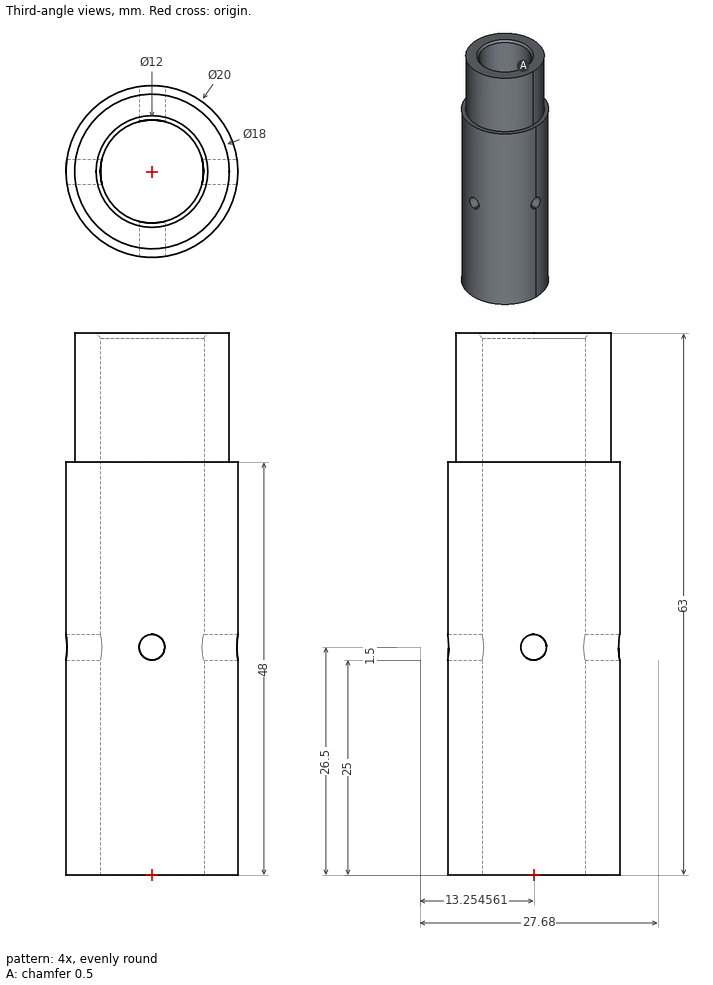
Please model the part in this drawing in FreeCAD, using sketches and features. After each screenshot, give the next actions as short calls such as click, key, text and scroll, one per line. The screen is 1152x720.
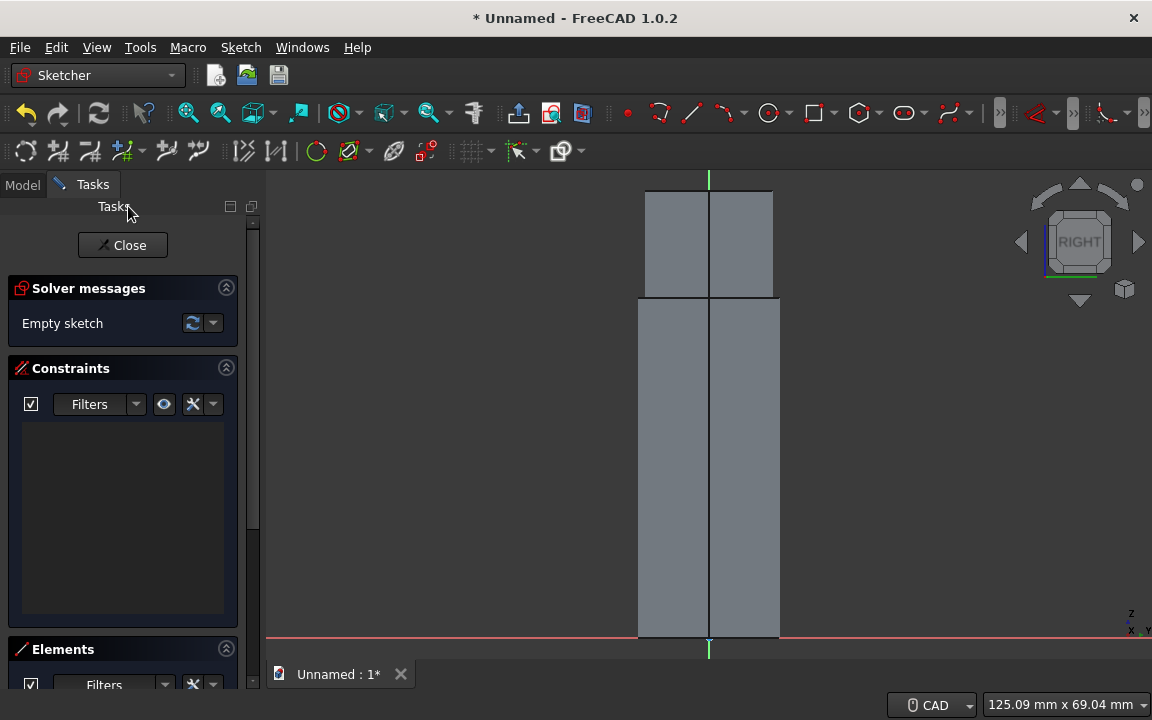
click(584, 114)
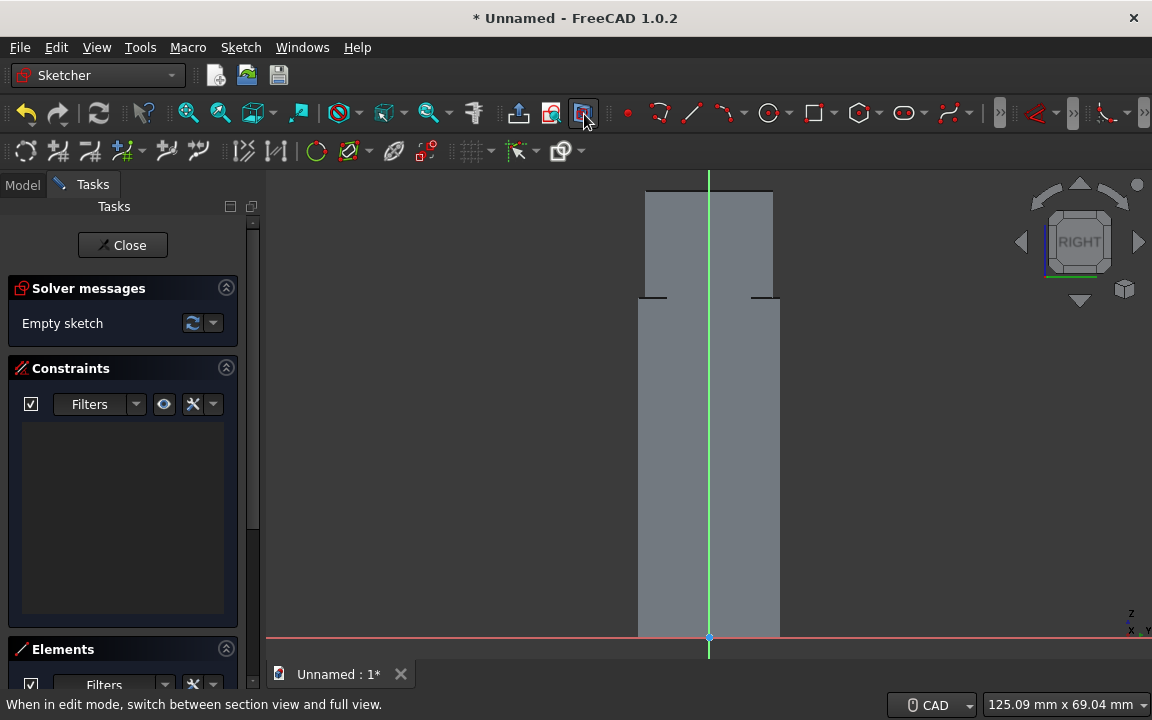
scroll(489, 198, down, 1)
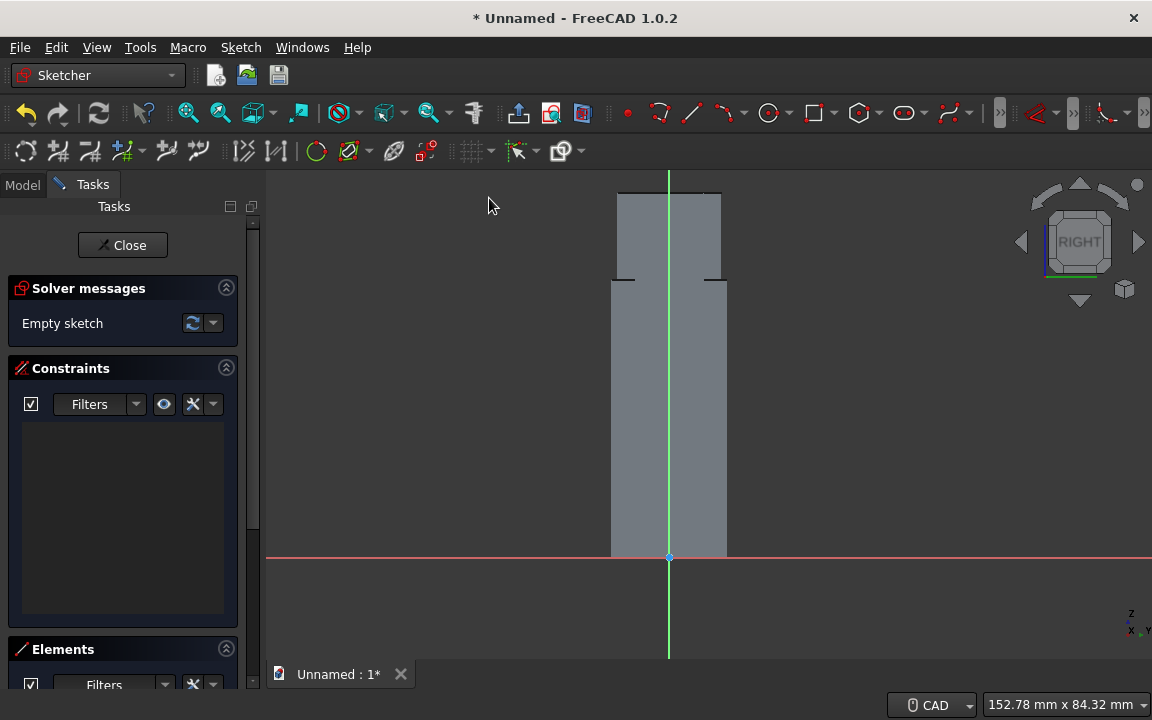
scroll(640, 562, up, 3)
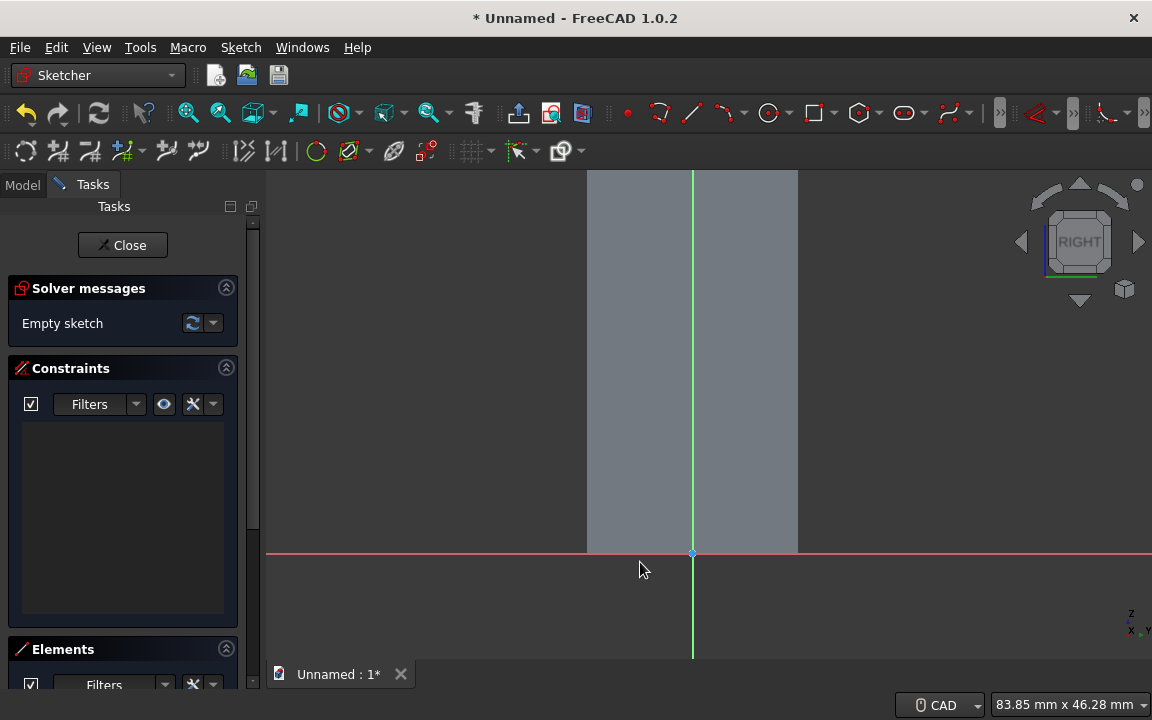
click(814, 114)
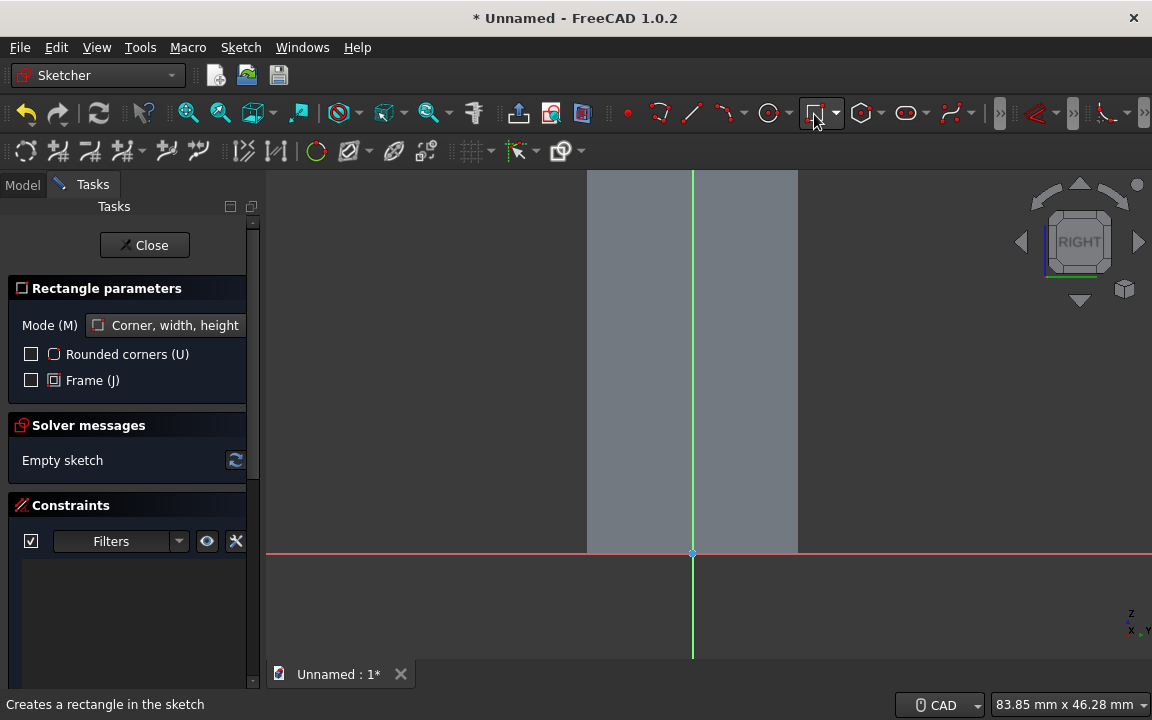
click(553, 274)
click(845, 290)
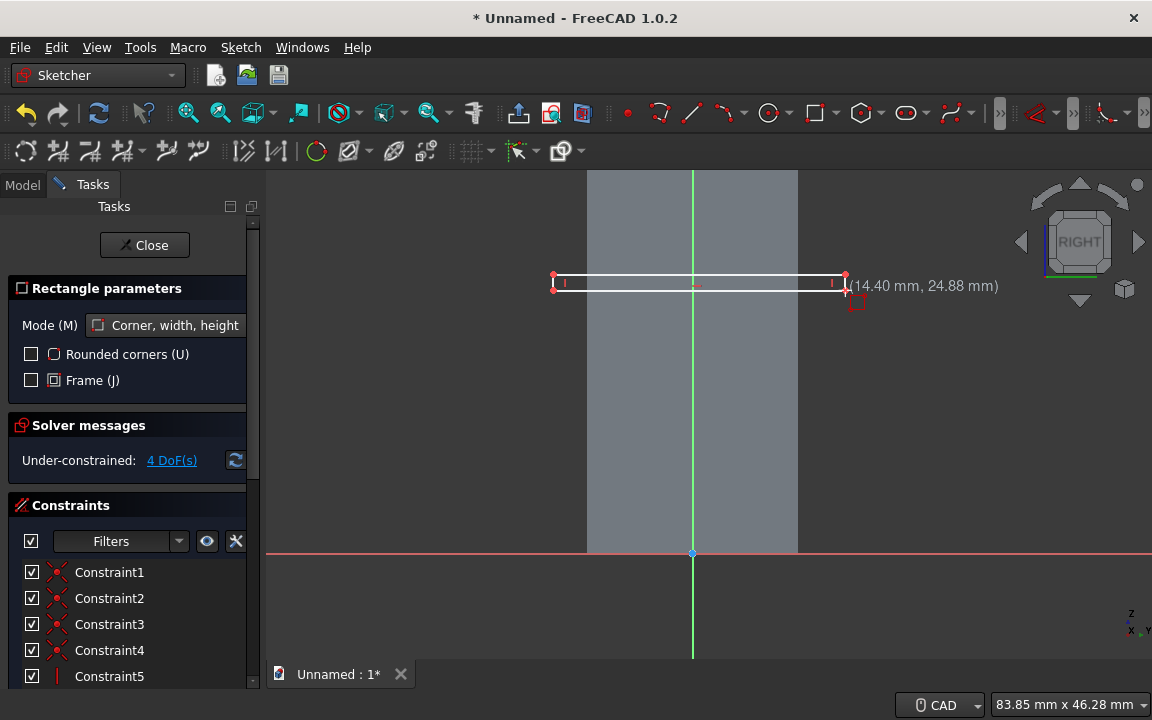
click(692, 114)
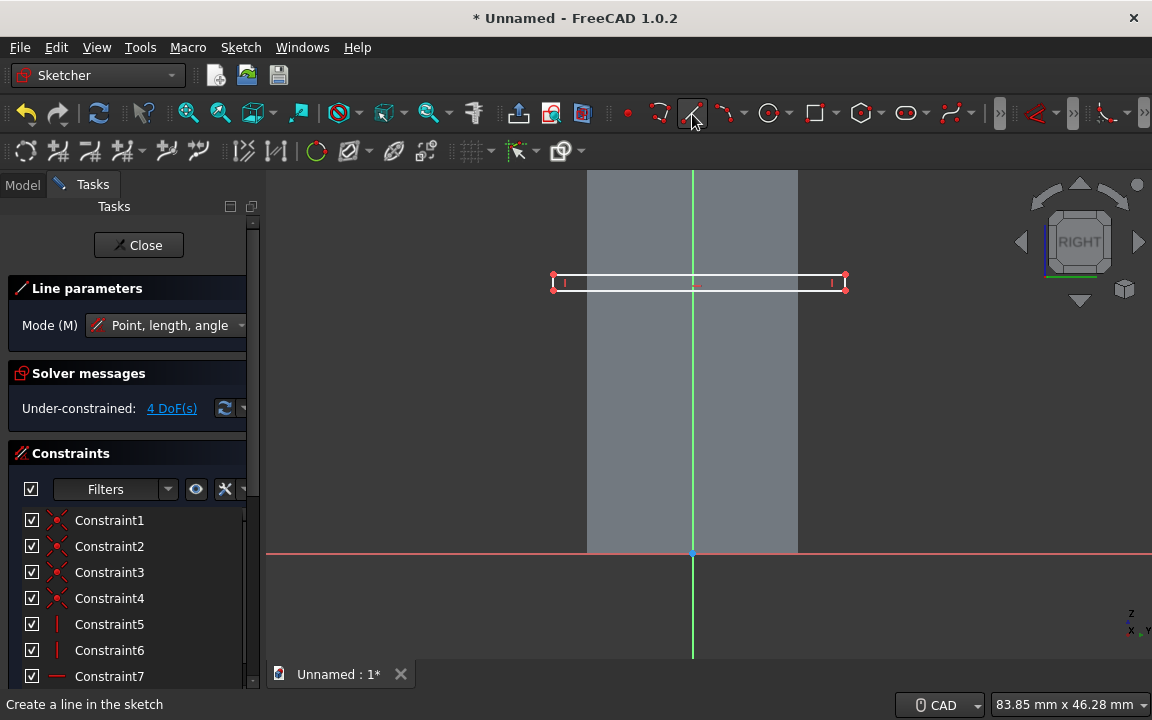
click(523, 274)
click(436, 274)
key(Escape)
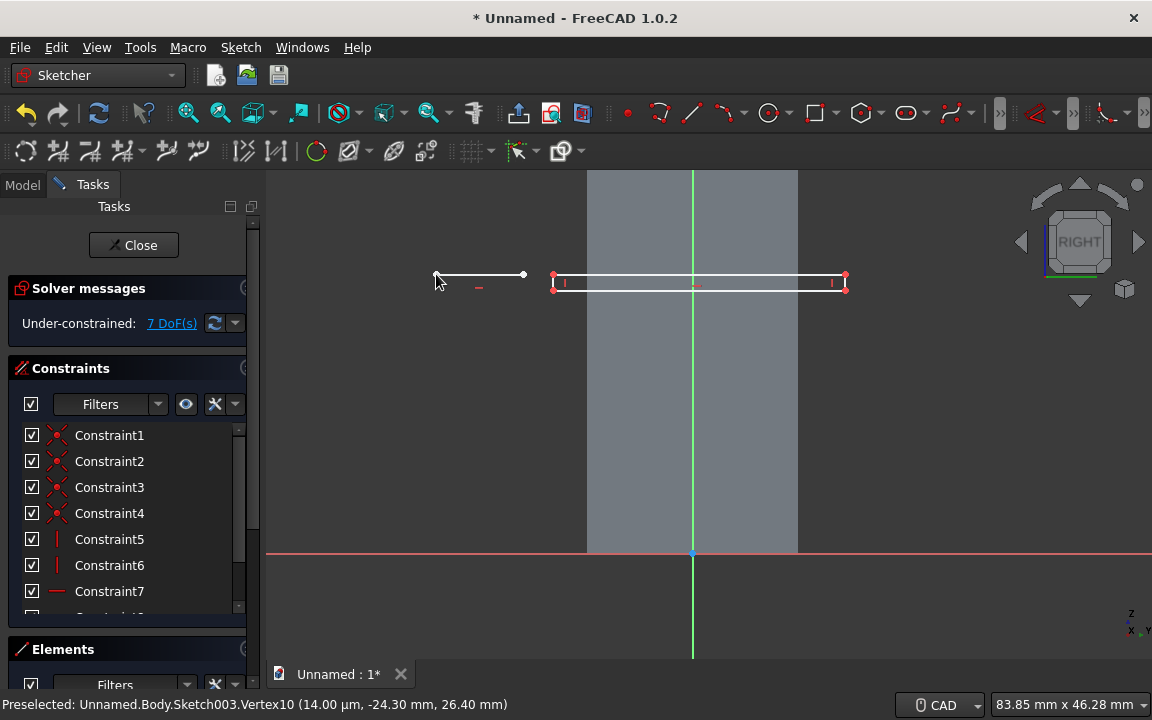
click(497, 275)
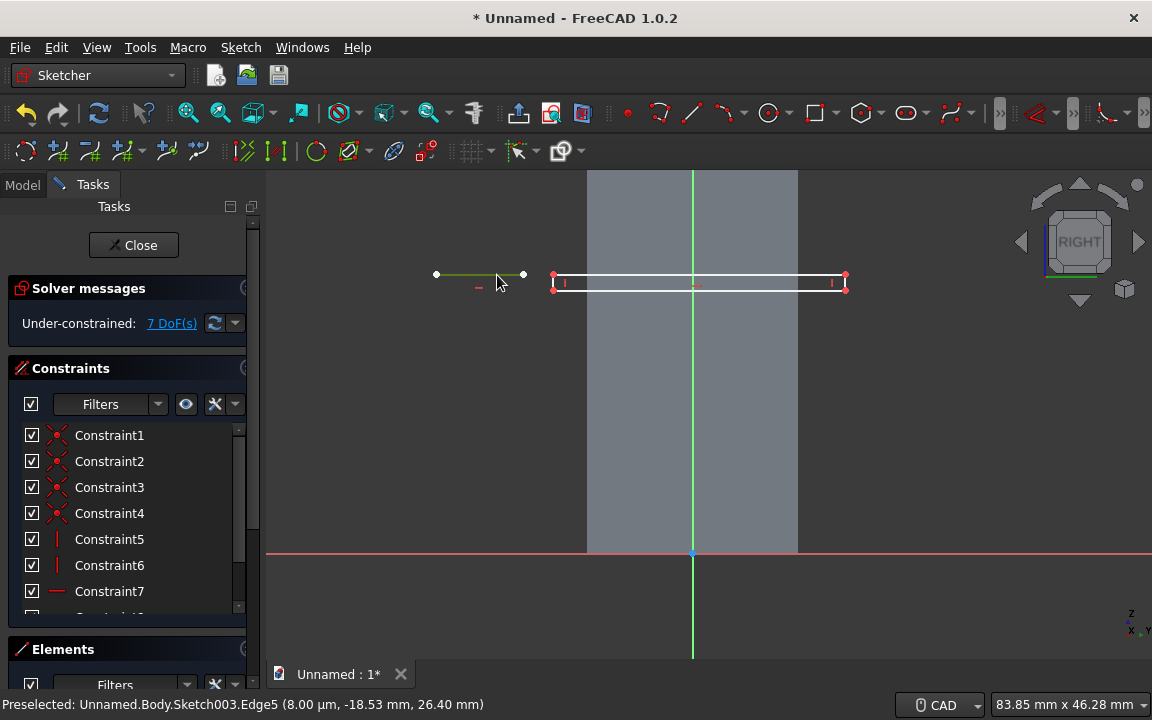
key(g)
key(n)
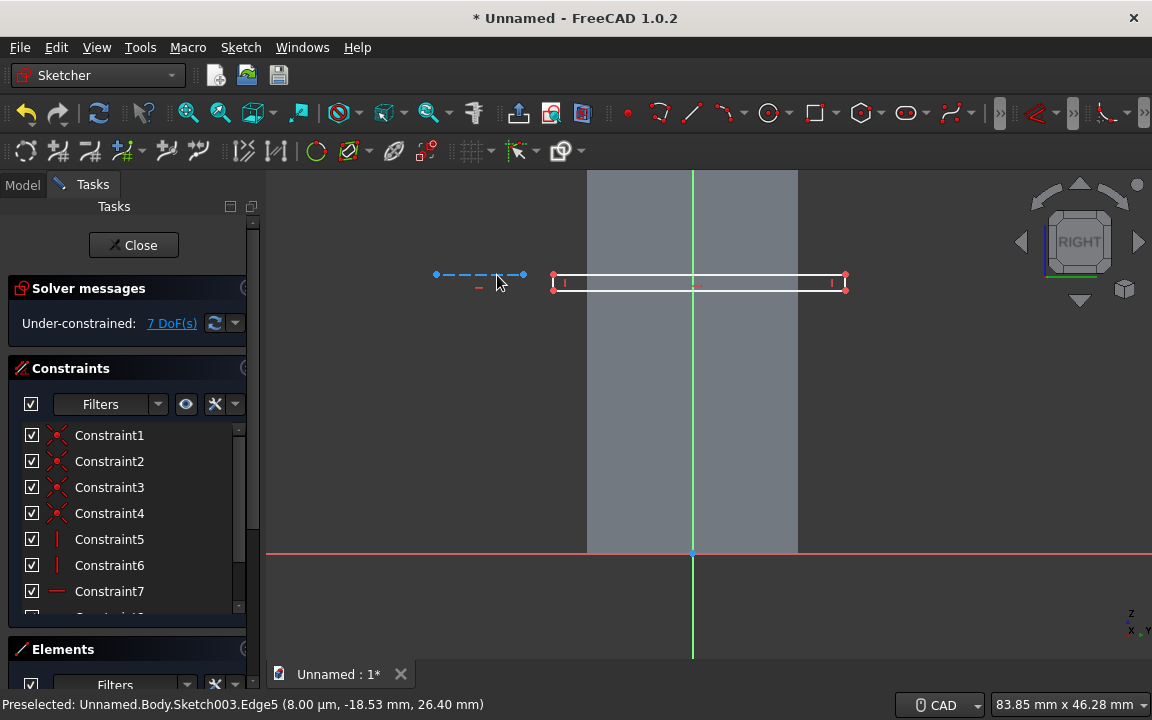
click(1036, 114)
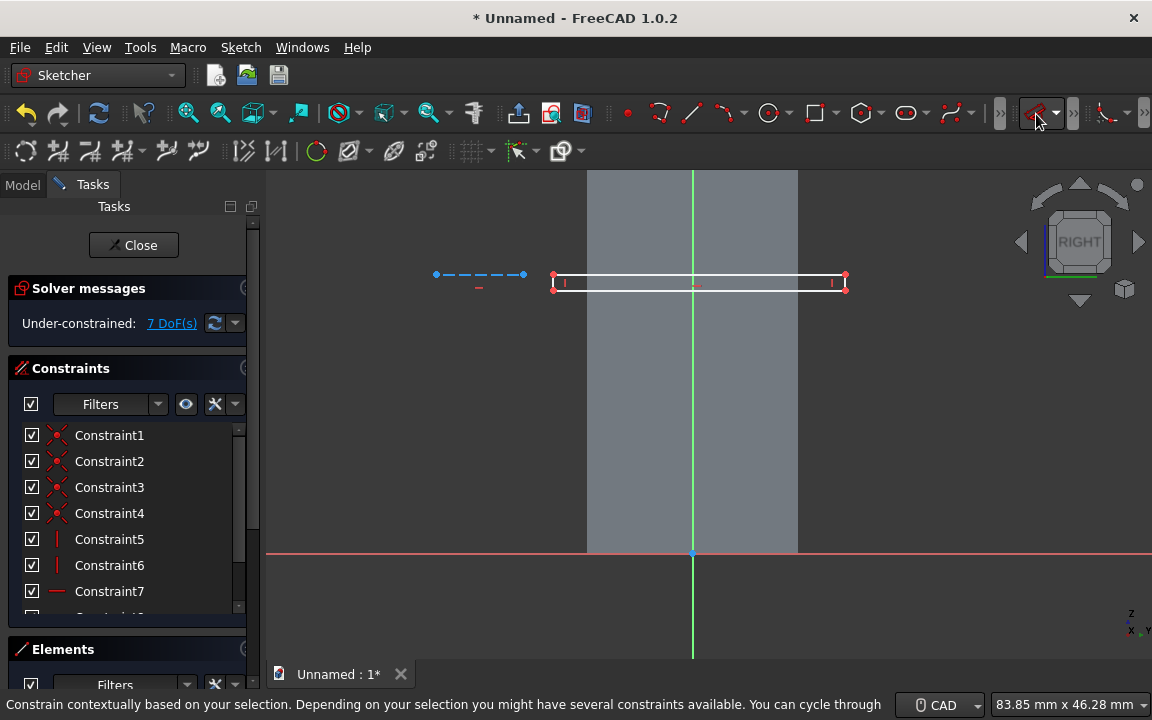
scroll(553, 283, up, 5)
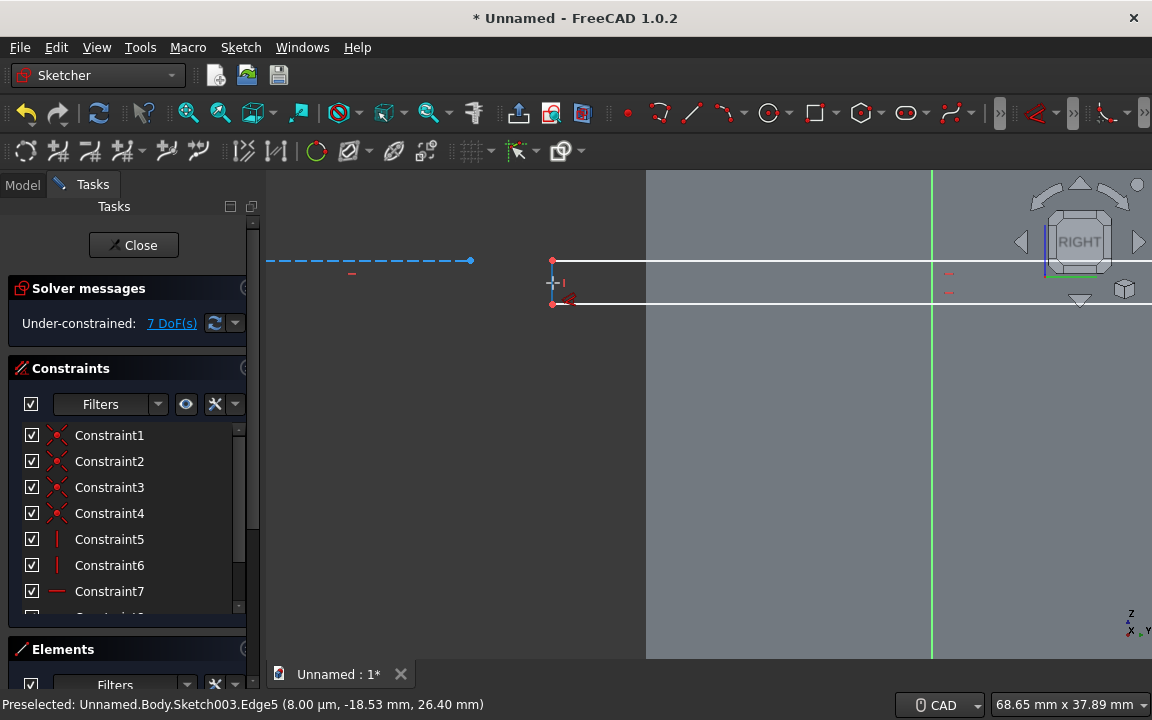
click(552, 283)
click(518, 283)